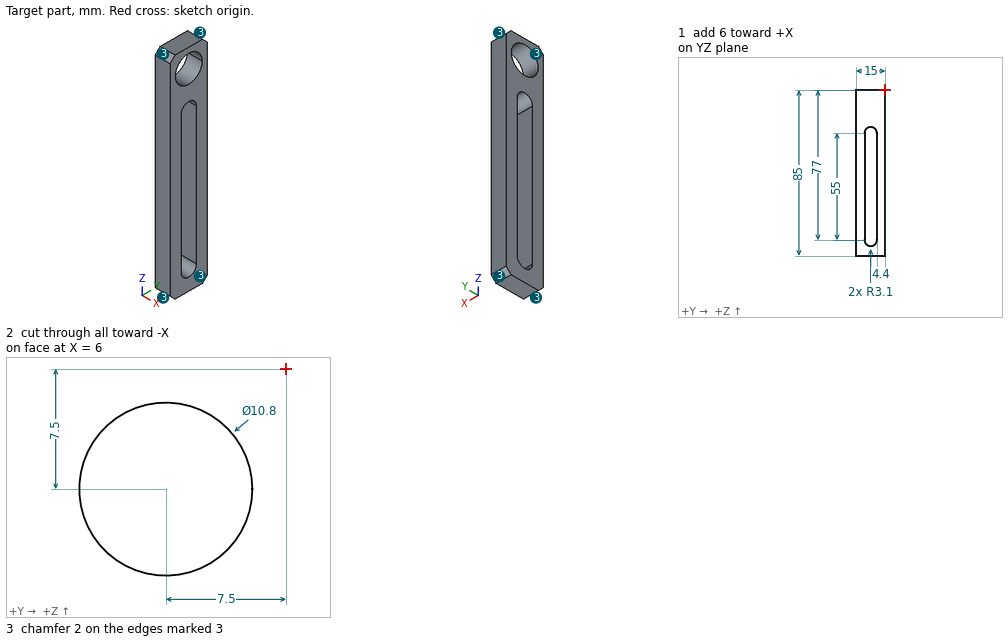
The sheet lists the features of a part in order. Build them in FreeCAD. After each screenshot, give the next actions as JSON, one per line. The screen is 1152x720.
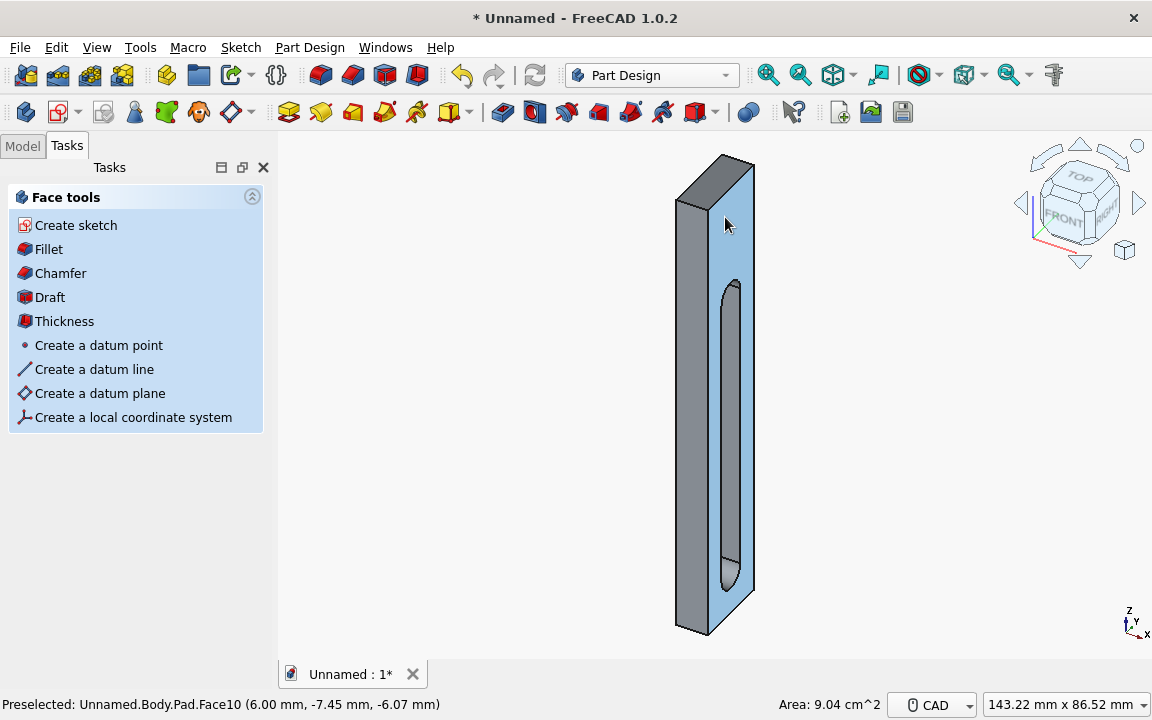
{"action": "left_click", "coordinate": [58, 112]}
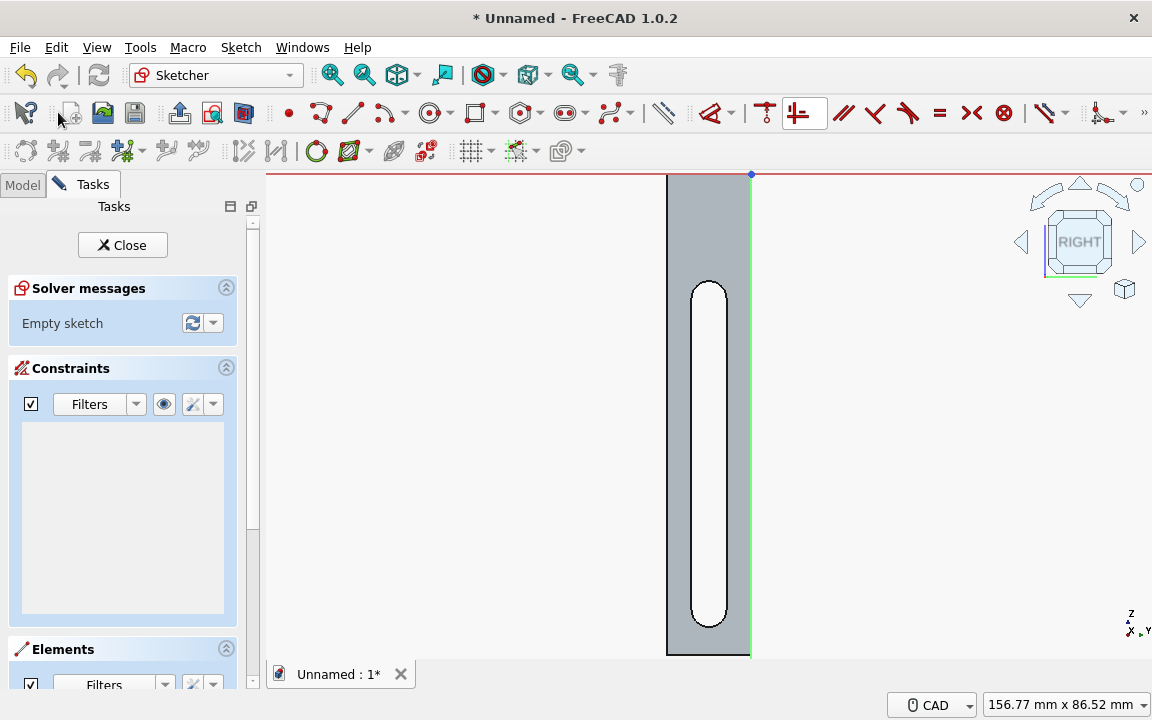
{"action": "scroll", "coordinate": [640, 414], "scroll_direction": "down", "scroll_amount": 5}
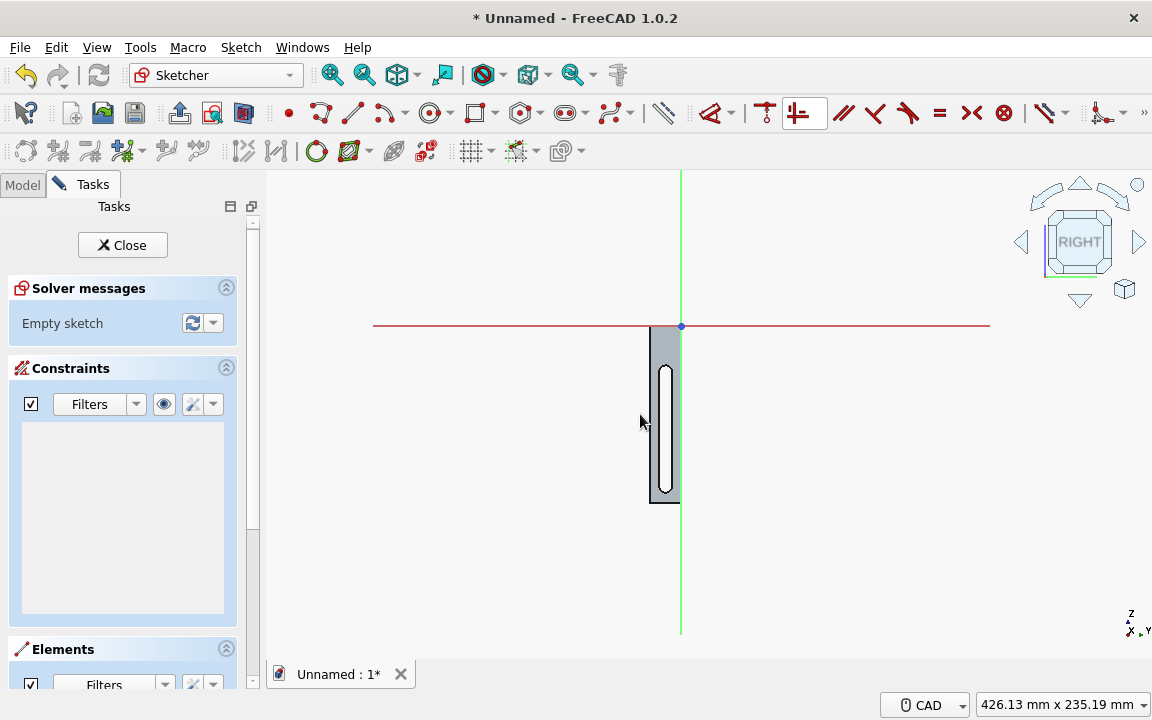
{"action": "scroll", "coordinate": [671, 332], "scroll_direction": "up", "scroll_amount": 12}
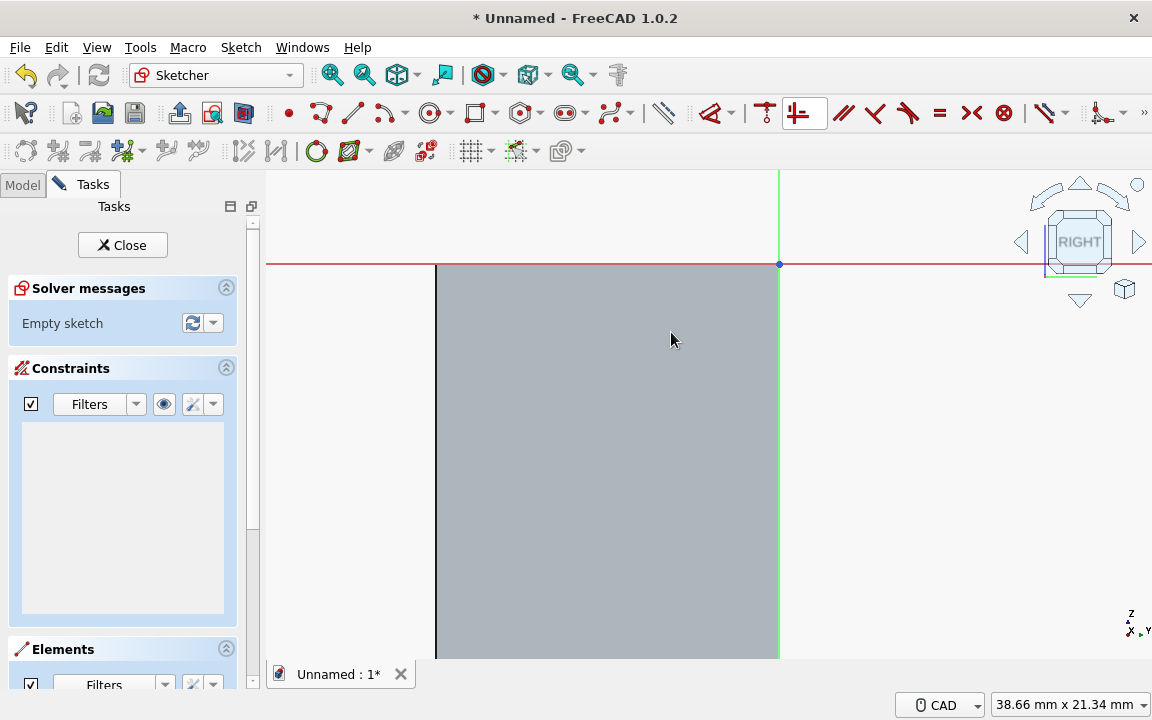
{"action": "left_click", "coordinate": [430, 114]}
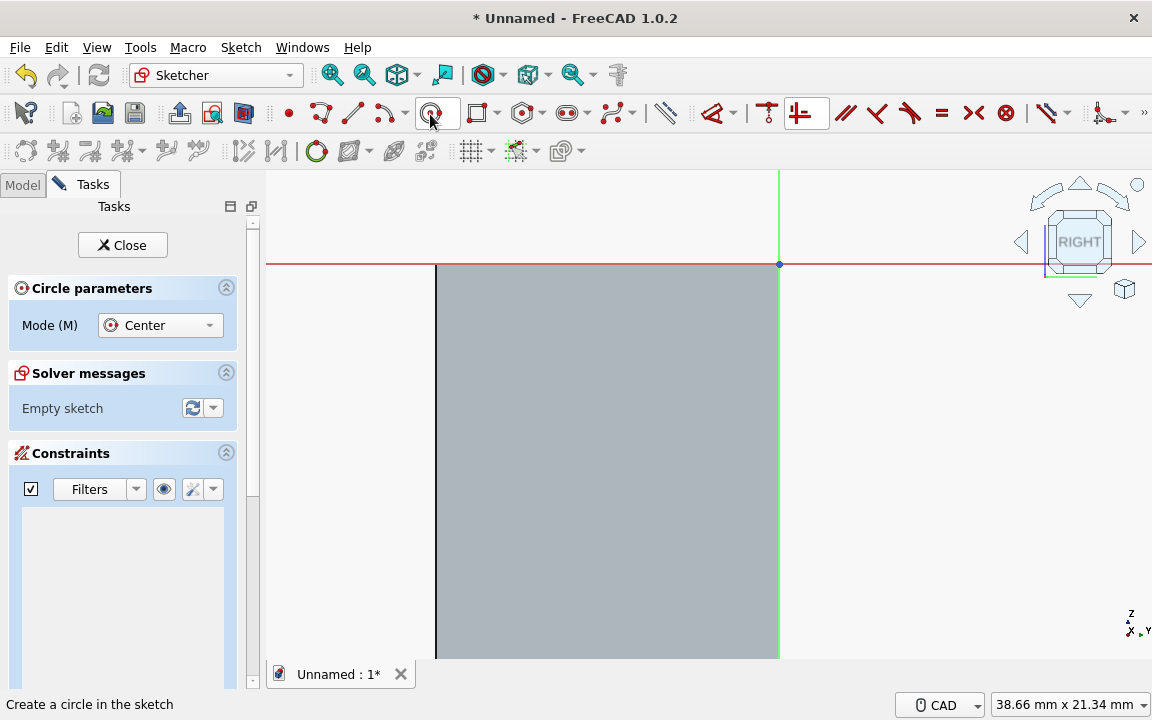
{"action": "left_click", "coordinate": [607, 436]}
{"action": "left_click", "coordinate": [695, 348]}
{"action": "key", "text": "Escape"}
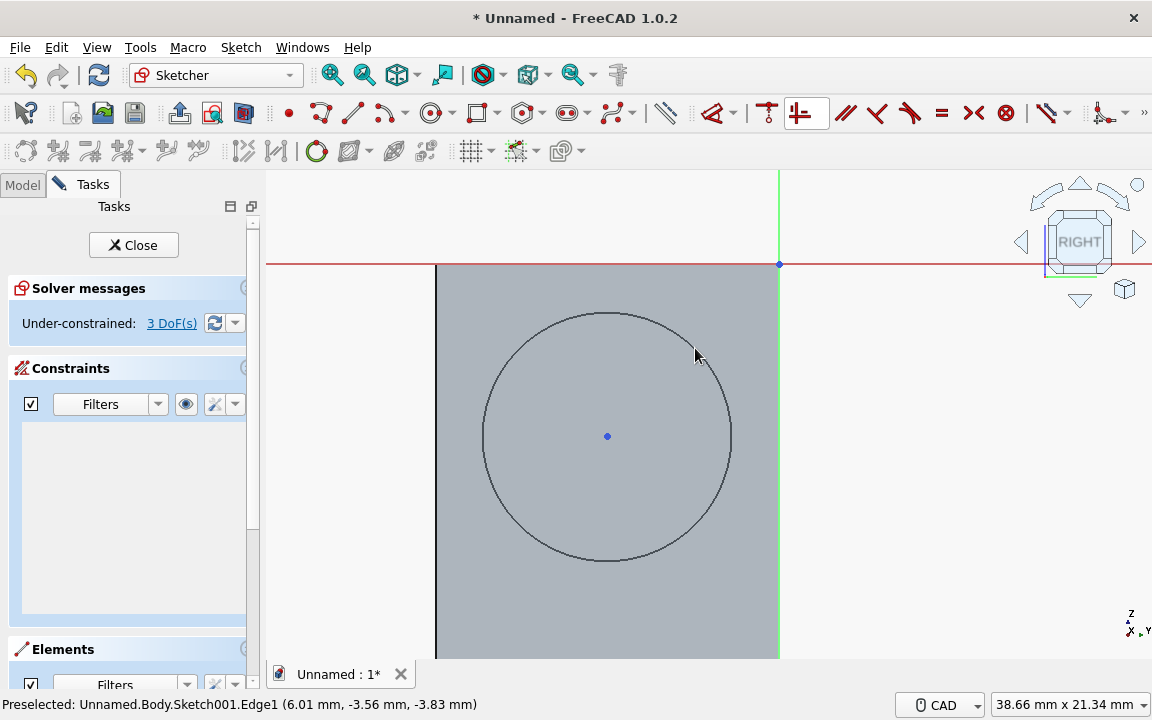
{"action": "left_click", "coordinate": [712, 114]}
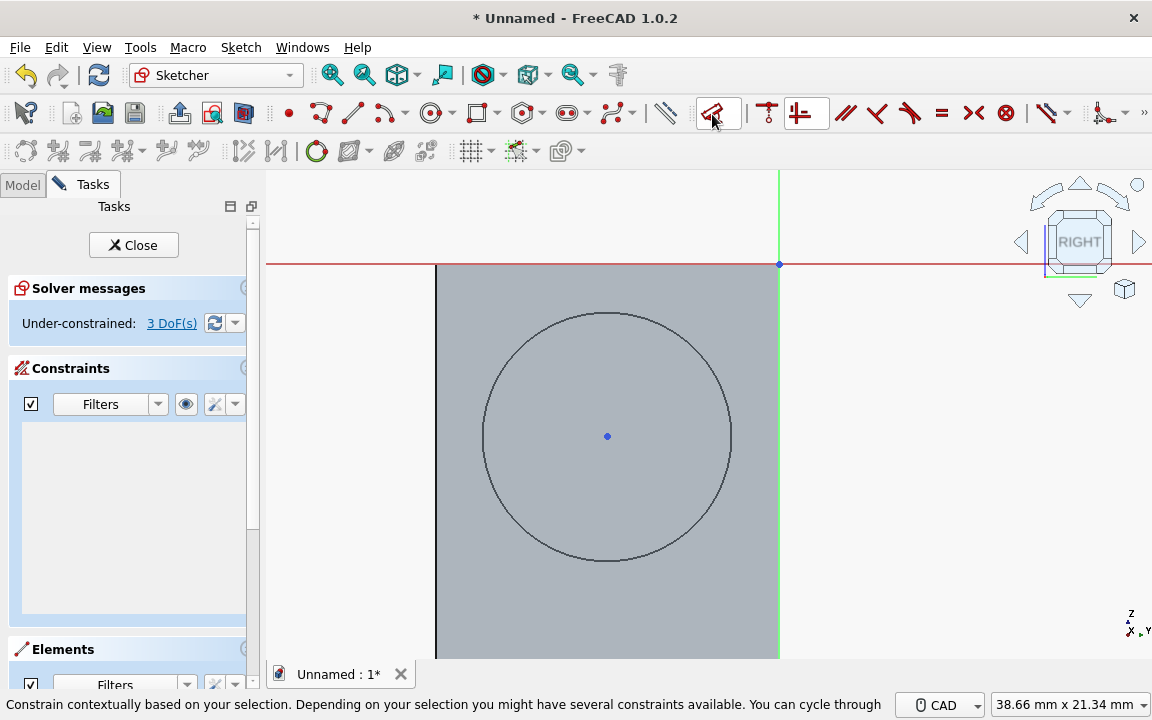
{"action": "left_click", "coordinate": [695, 349]}
{"action": "left_click", "coordinate": [718, 326]}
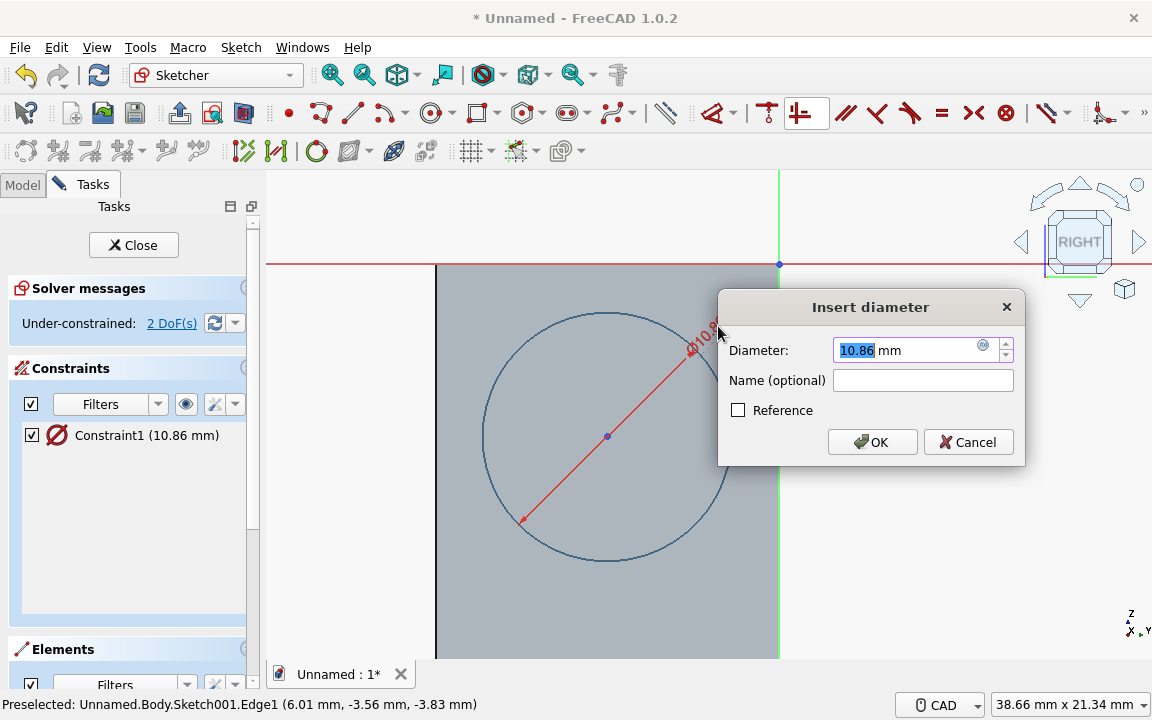
{"action": "type", "text": "10.8"}
{"action": "key", "text": "Return"}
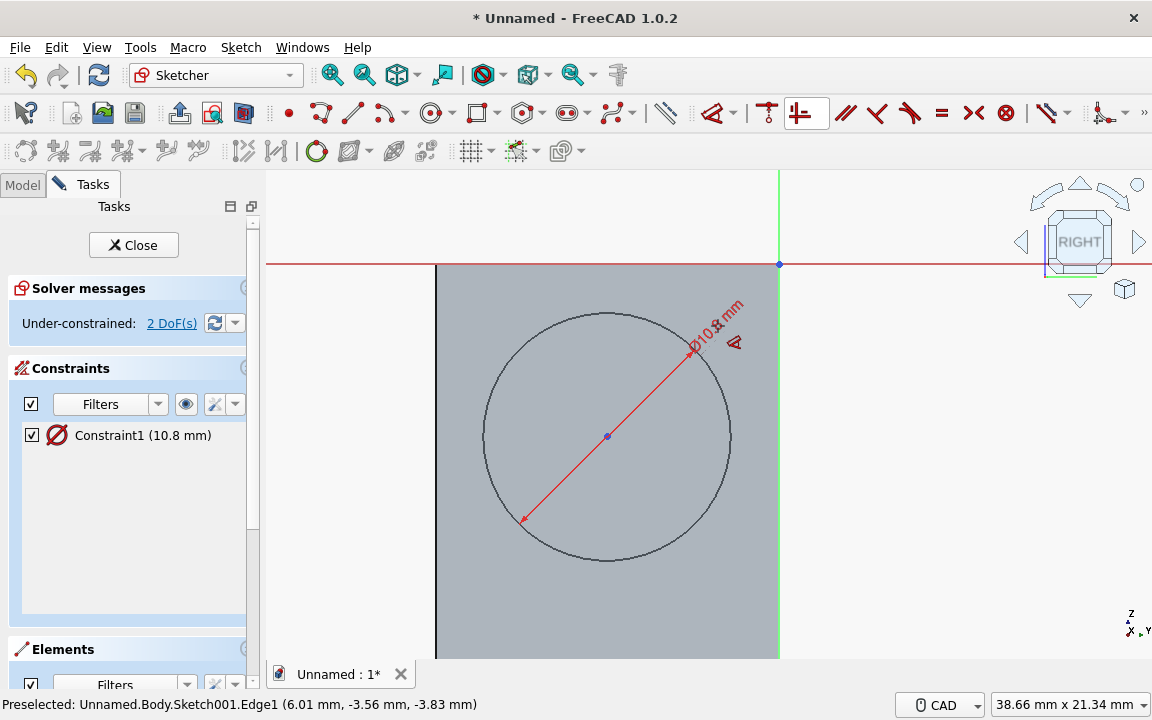
{"action": "left_click", "coordinate": [607, 437]}
{"action": "left_click", "coordinate": [693, 230]}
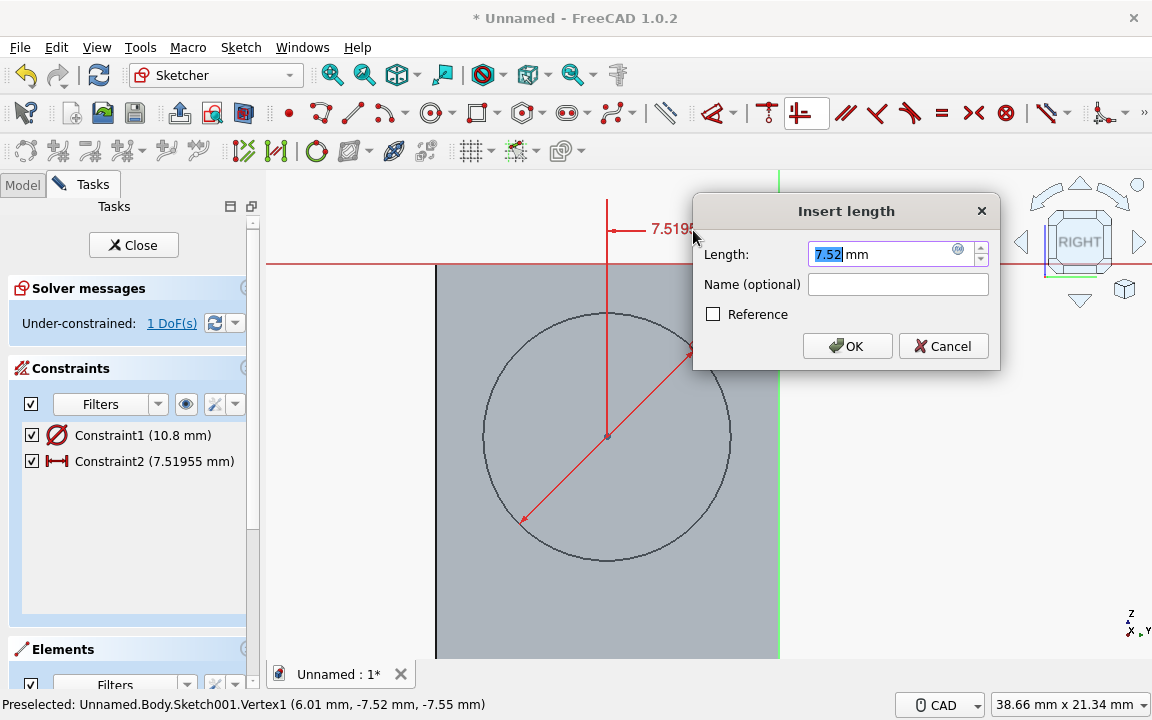
{"action": "type", "text": "7.5"}
{"action": "key", "text": "Return"}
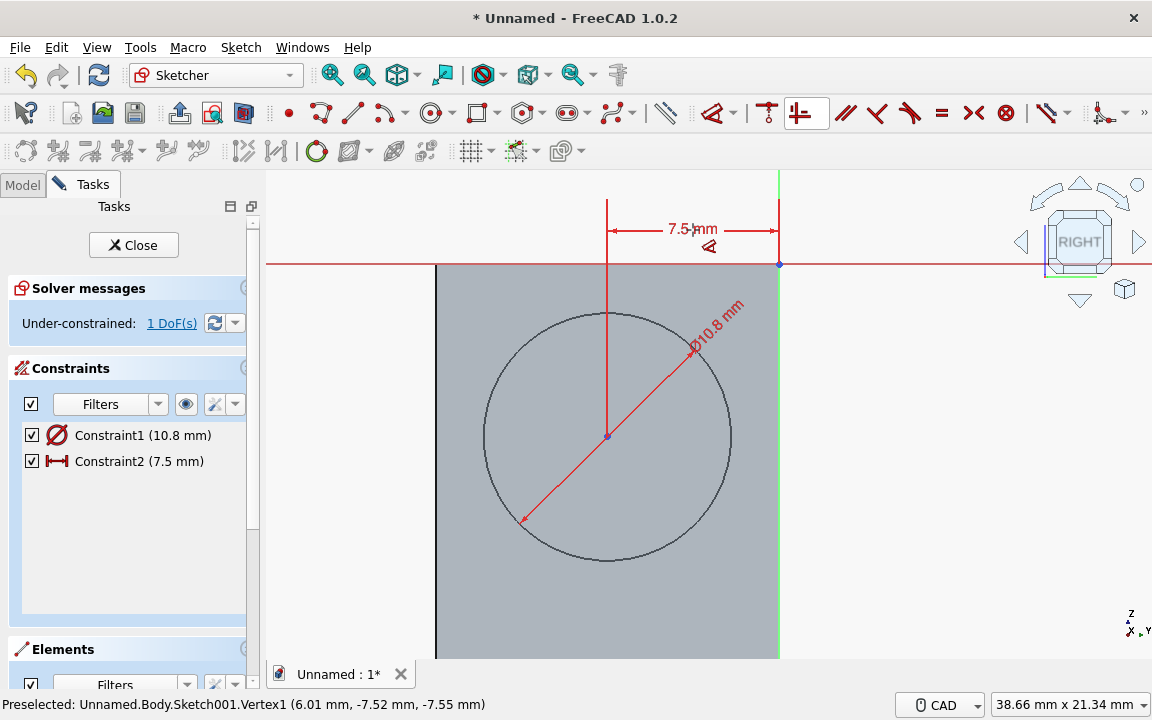
{"action": "left_click", "coordinate": [607, 437]}
{"action": "left_click", "coordinate": [813, 351]}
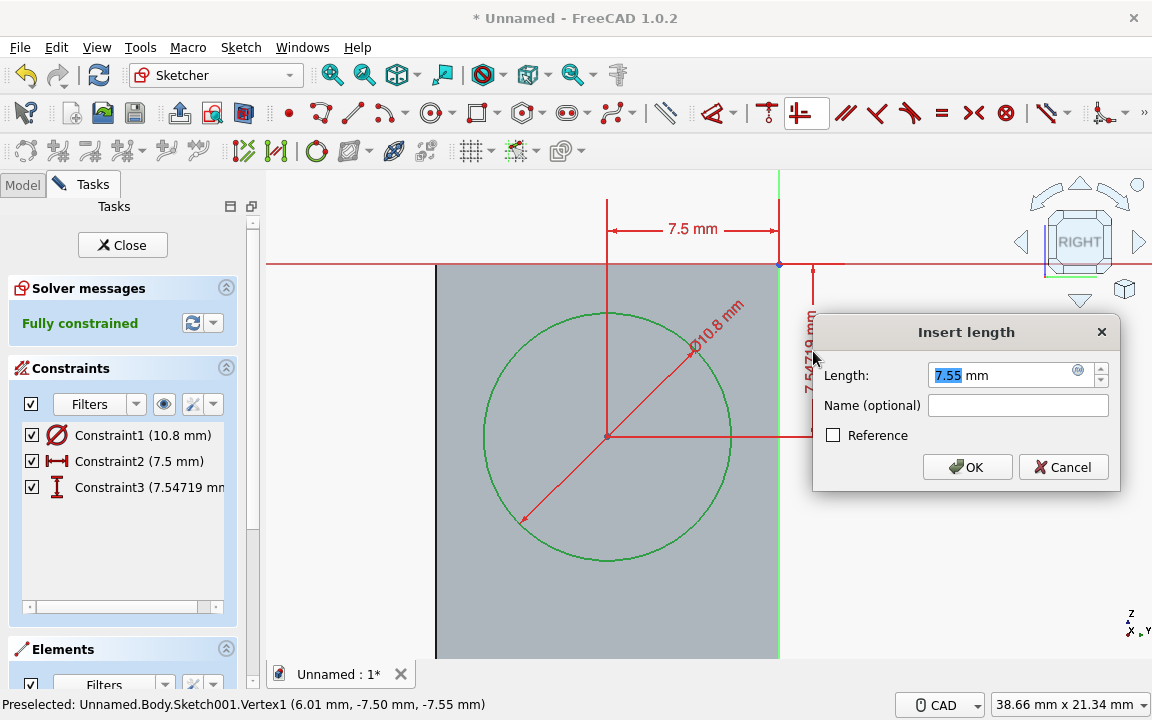
{"action": "type", "text": "7.5"}
{"action": "key", "text": "Return"}
{"action": "key", "text": "Escape"}